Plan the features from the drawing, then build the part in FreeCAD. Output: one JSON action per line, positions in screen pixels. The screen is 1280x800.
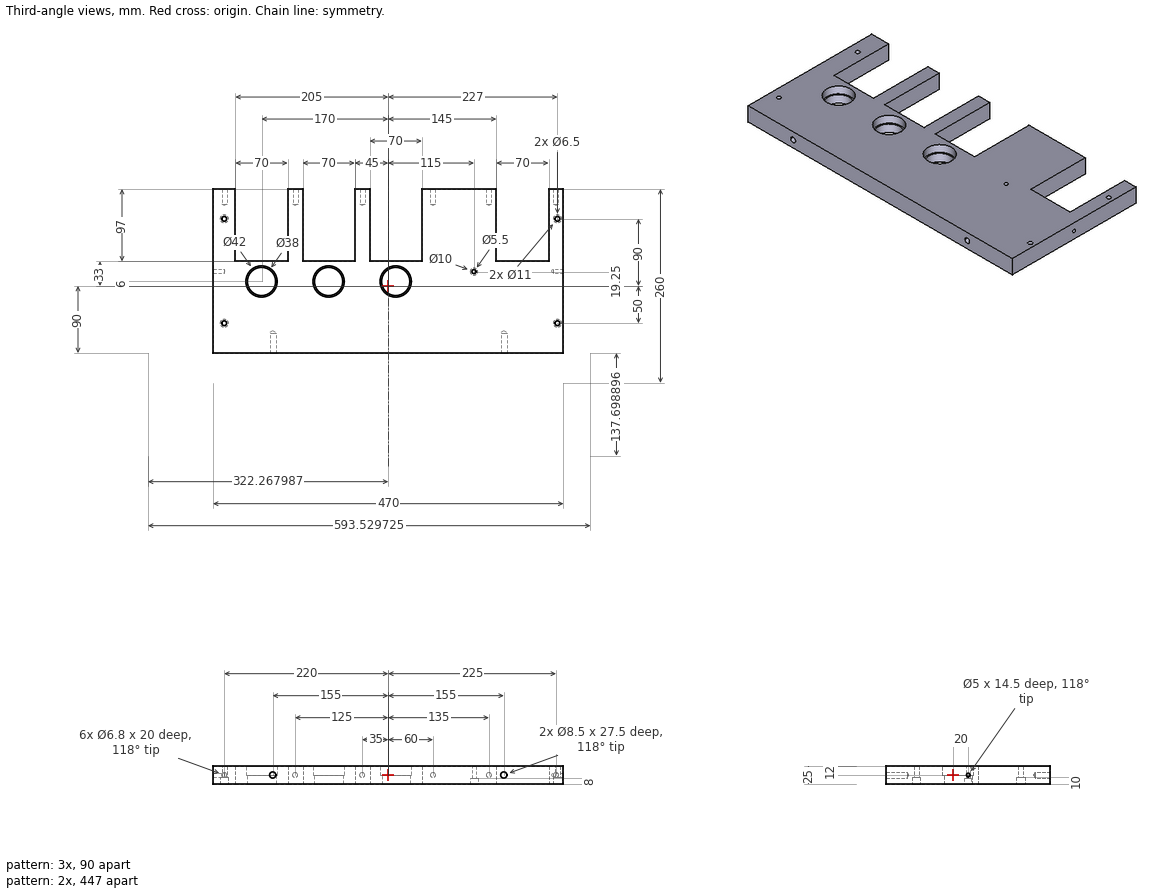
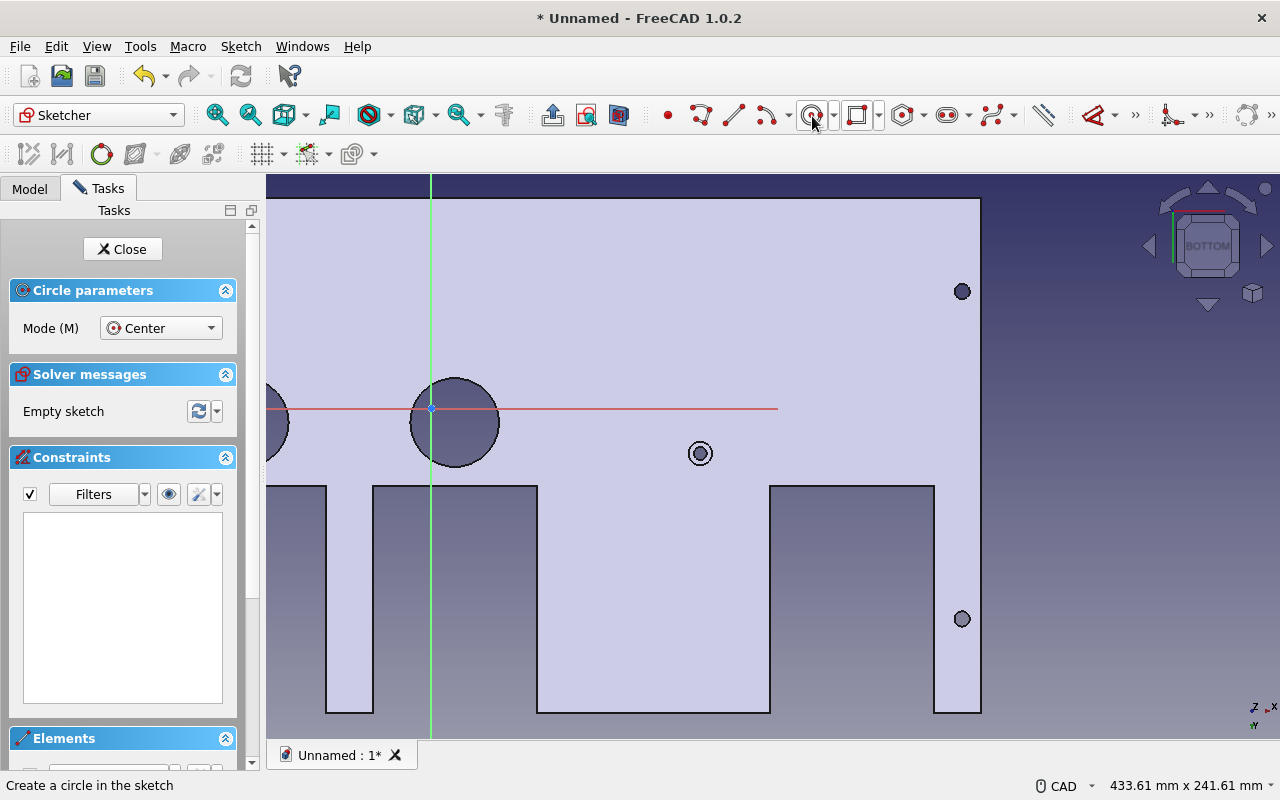
{"action": "scroll", "coordinate": [962, 619], "scroll_direction": "up", "scroll_amount": 3}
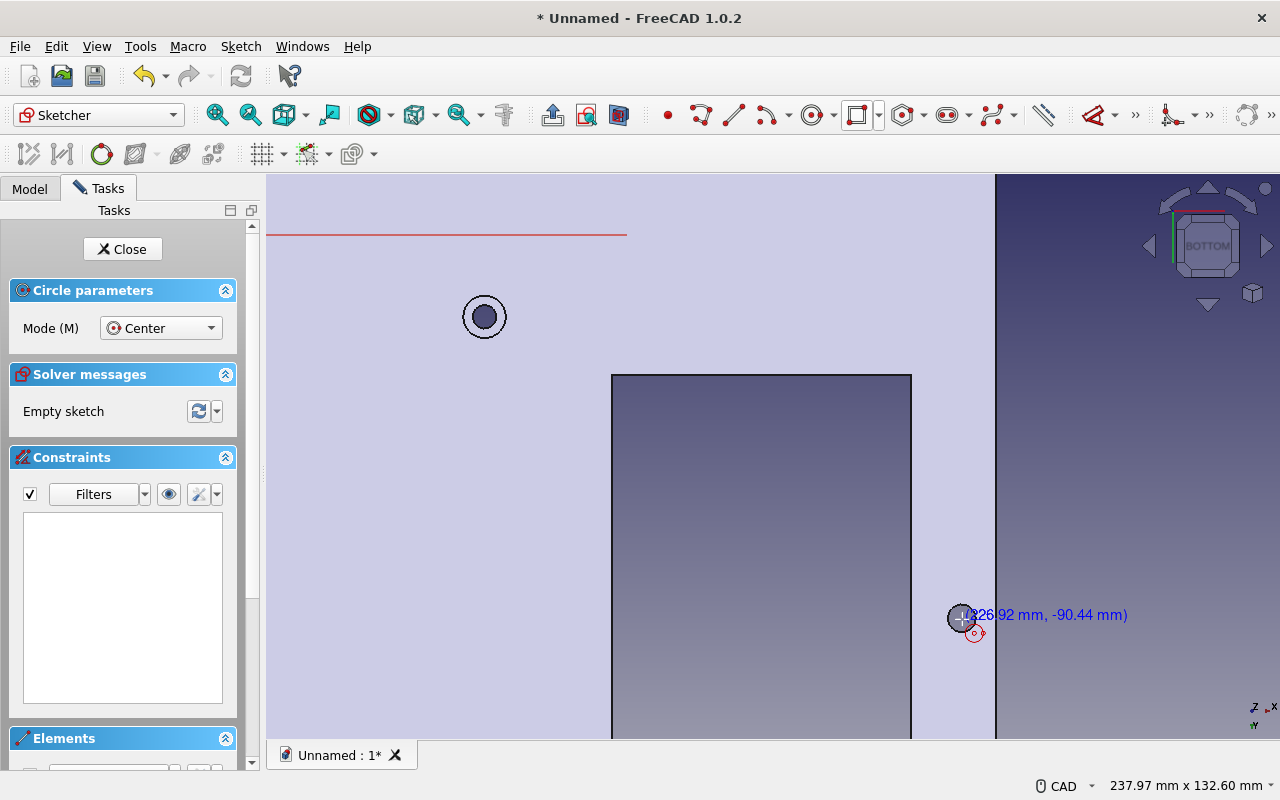
{"action": "left_click", "coordinate": [962, 618]}
{"action": "mouse_move", "coordinate": [978, 602]}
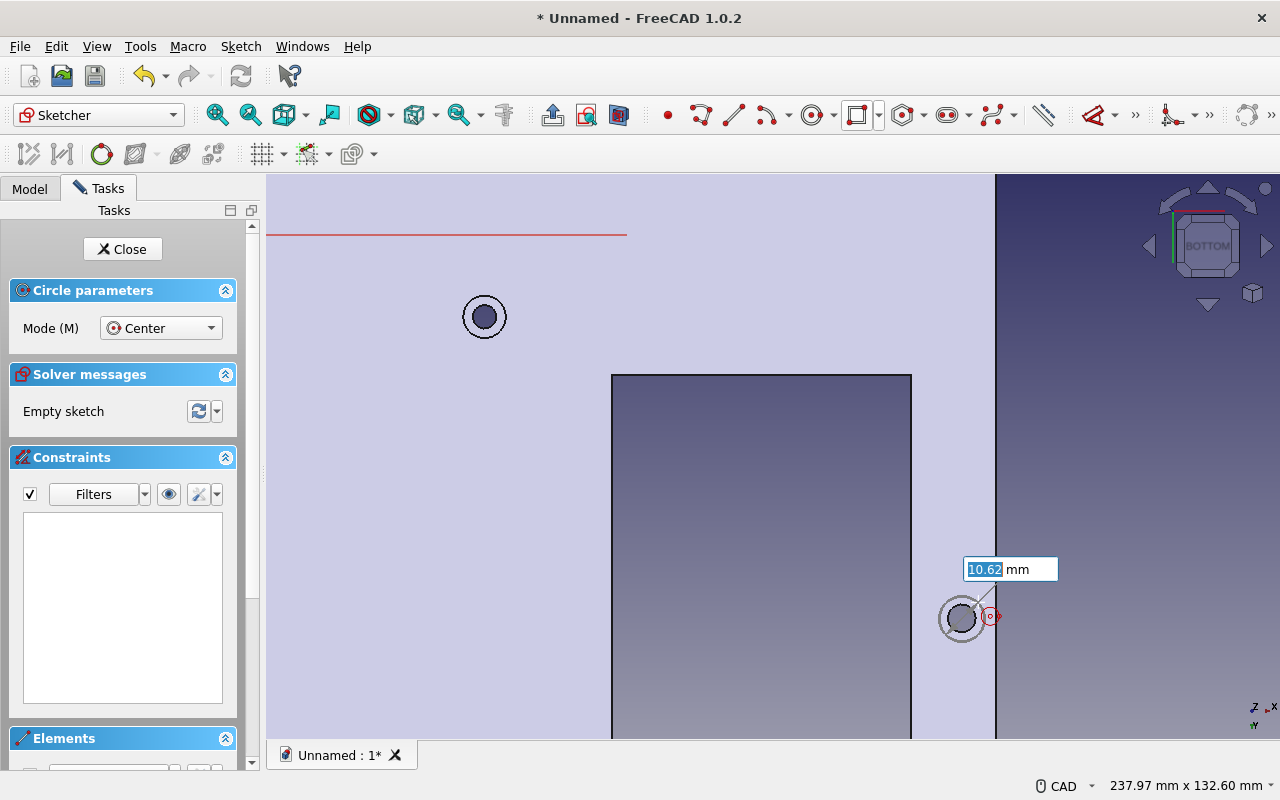
{"action": "type", "text": "11"}
{"action": "key", "text": "Return"}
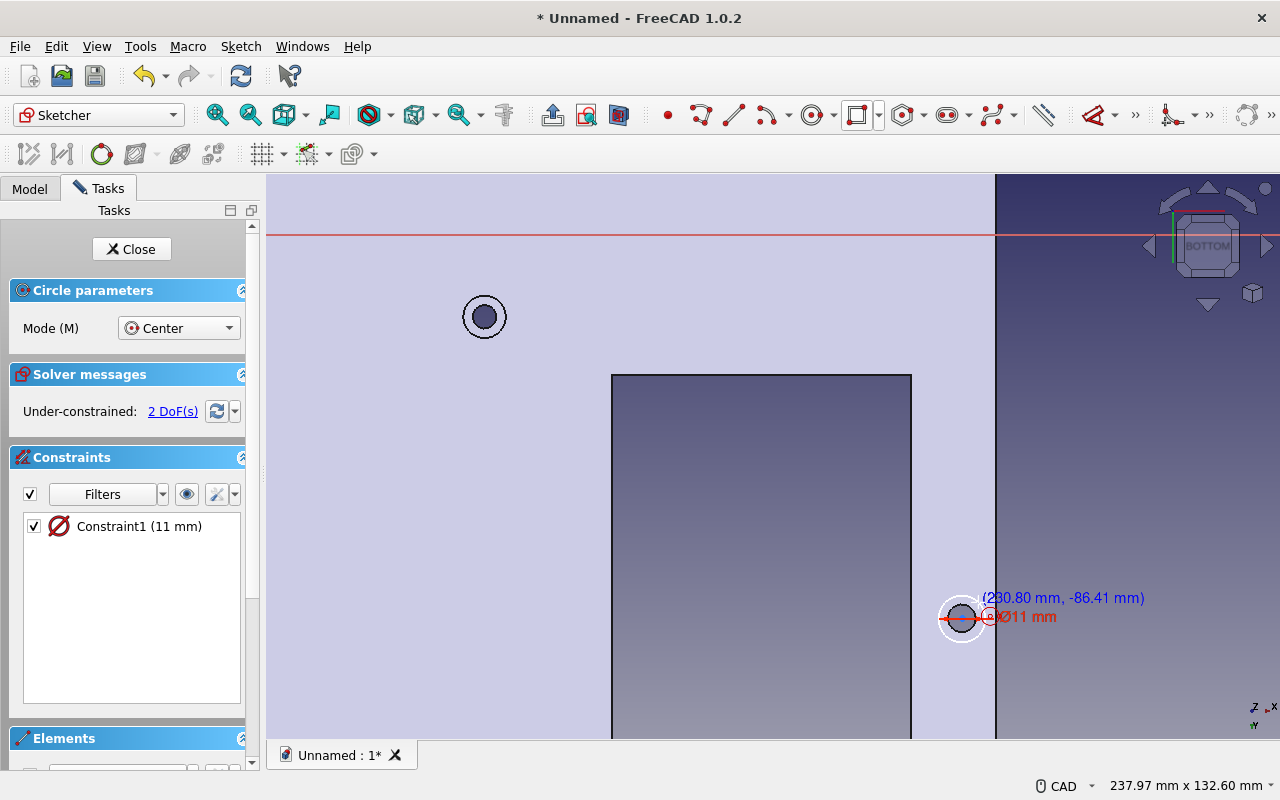
{"action": "scroll", "coordinate": [966, 623], "scroll_direction": "down", "scroll_amount": 3}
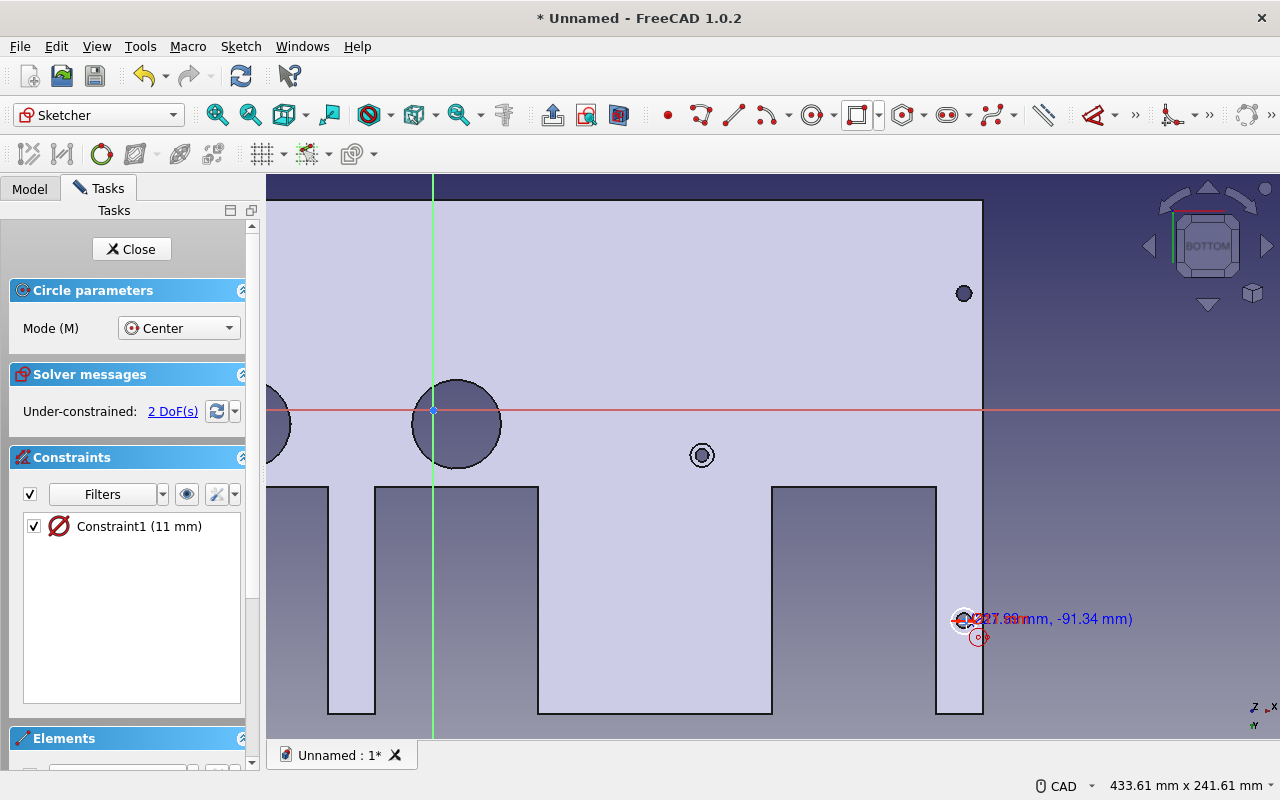
{"action": "scroll", "coordinate": [964, 293], "scroll_direction": "up", "scroll_amount": 3}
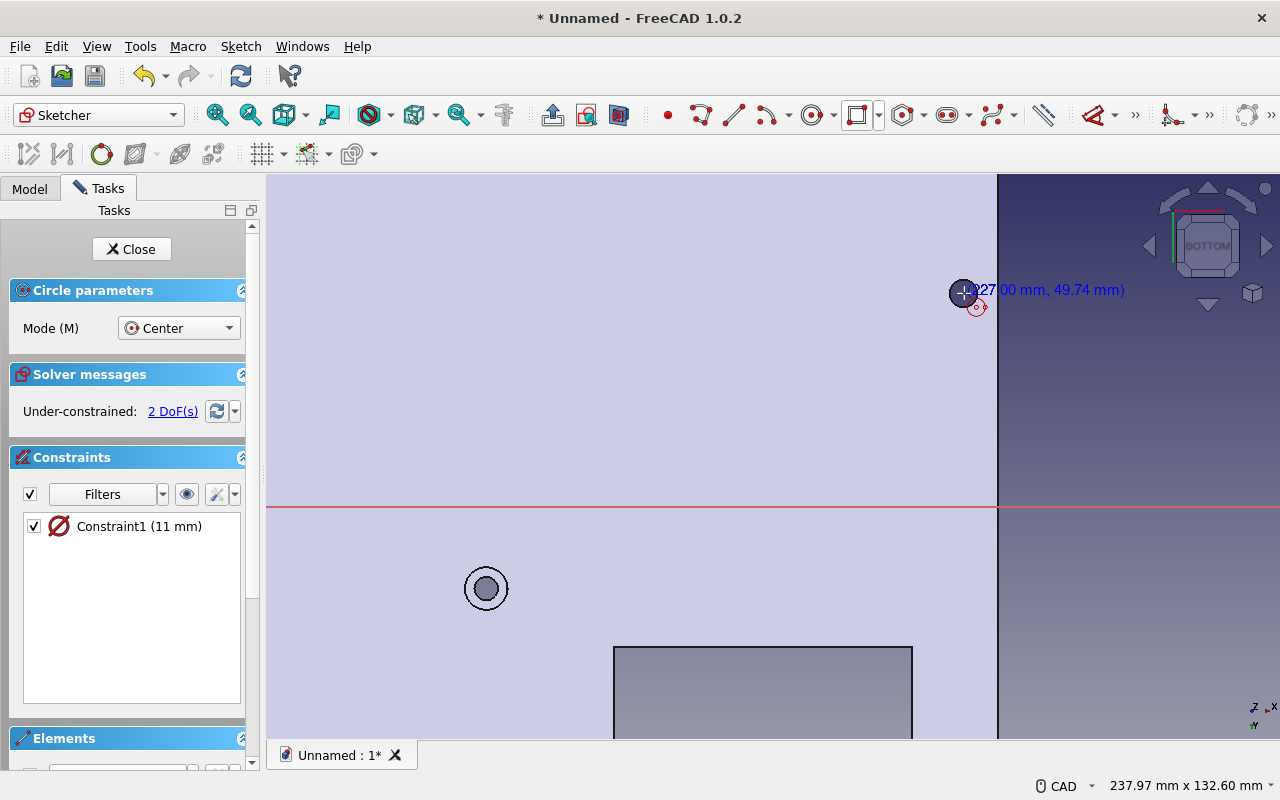
{"action": "left_click", "coordinate": [963, 294]}
{"action": "mouse_move", "coordinate": [980, 277]}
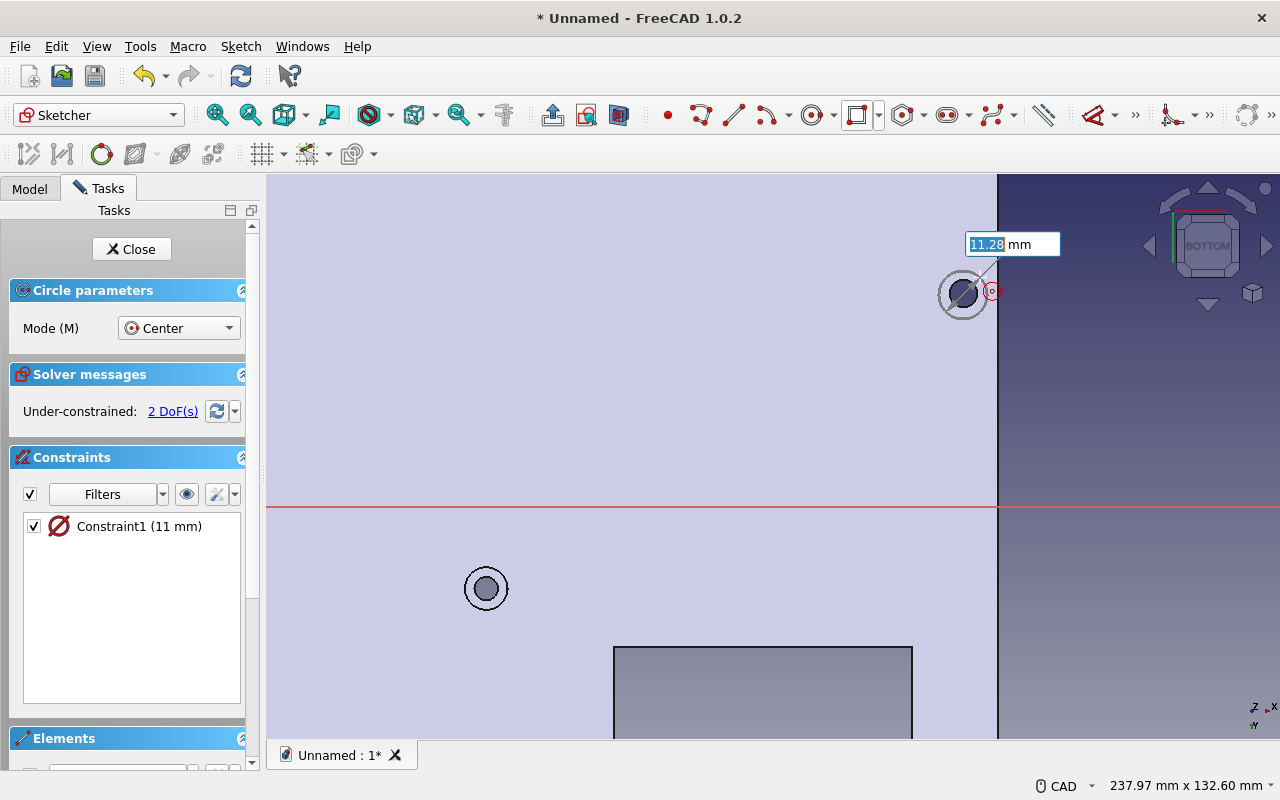
{"action": "type", "text": "11"}
{"action": "key", "text": "Return"}
{"action": "key", "text": "Escape"}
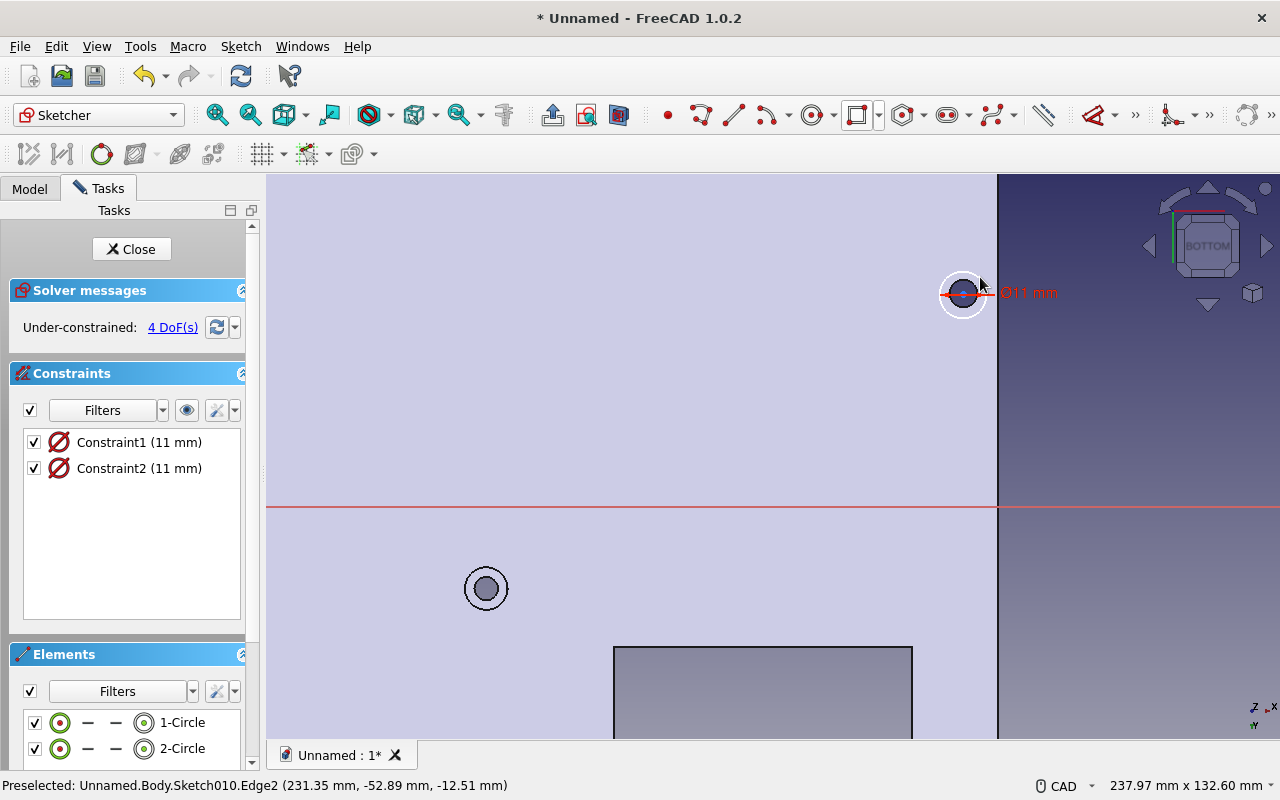
{"action": "left_click", "coordinate": [1092, 116]}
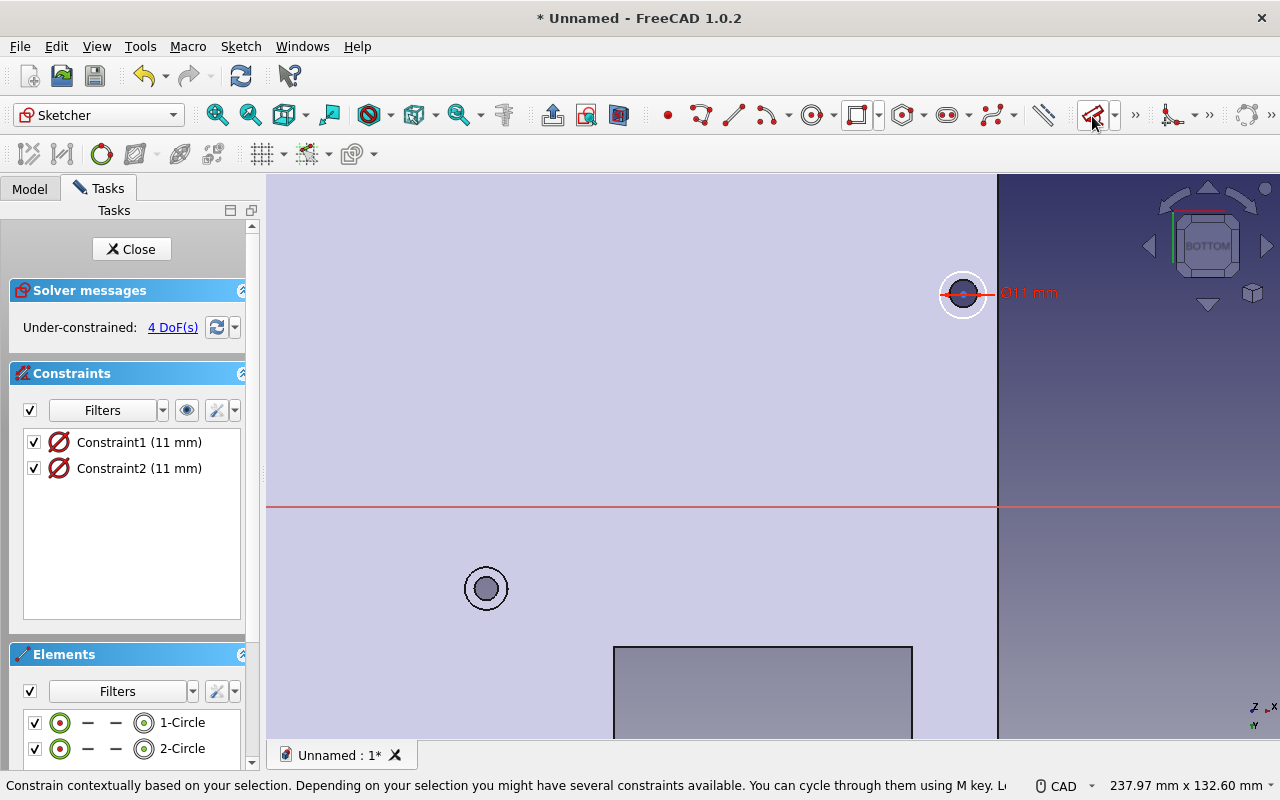
{"action": "scroll", "coordinate": [964, 292], "scroll_direction": "down", "scroll_amount": 3}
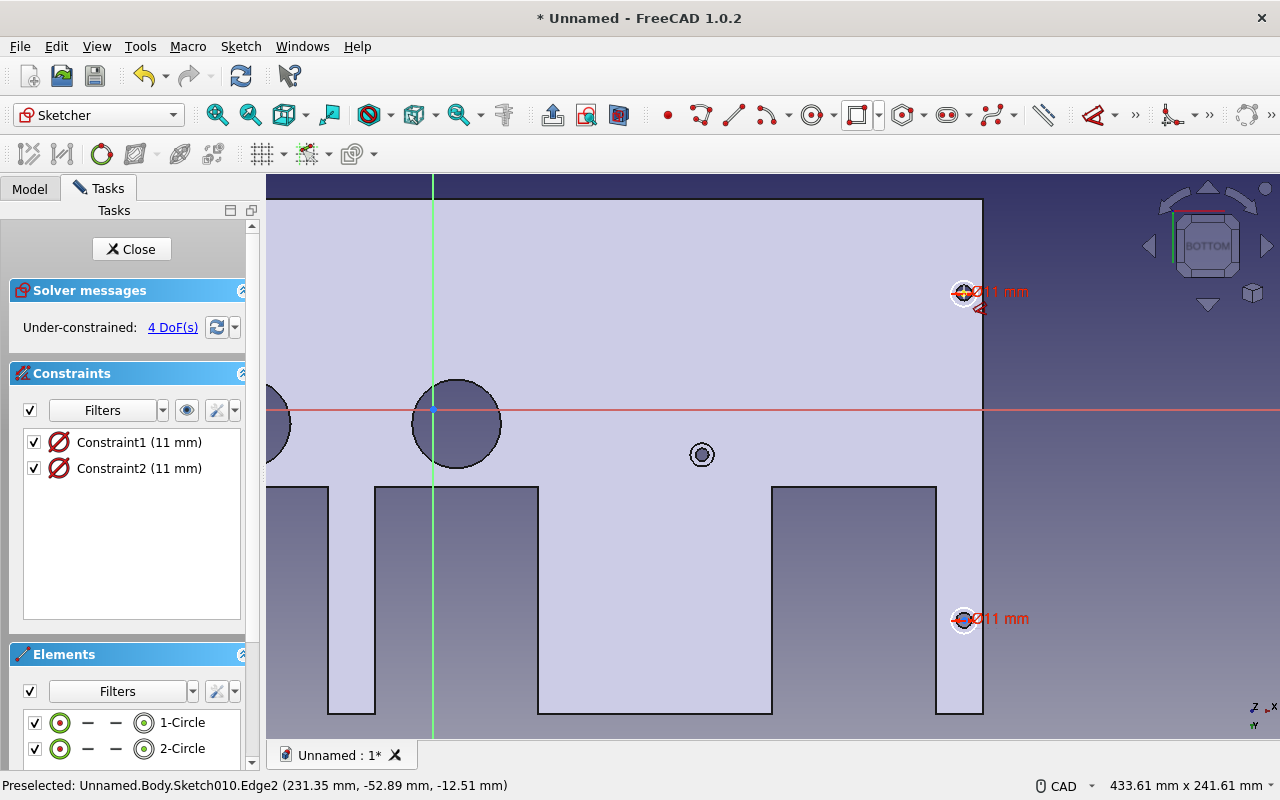
{"action": "left_click", "coordinate": [964, 621]}
{"action": "left_click", "coordinate": [399, 515]}